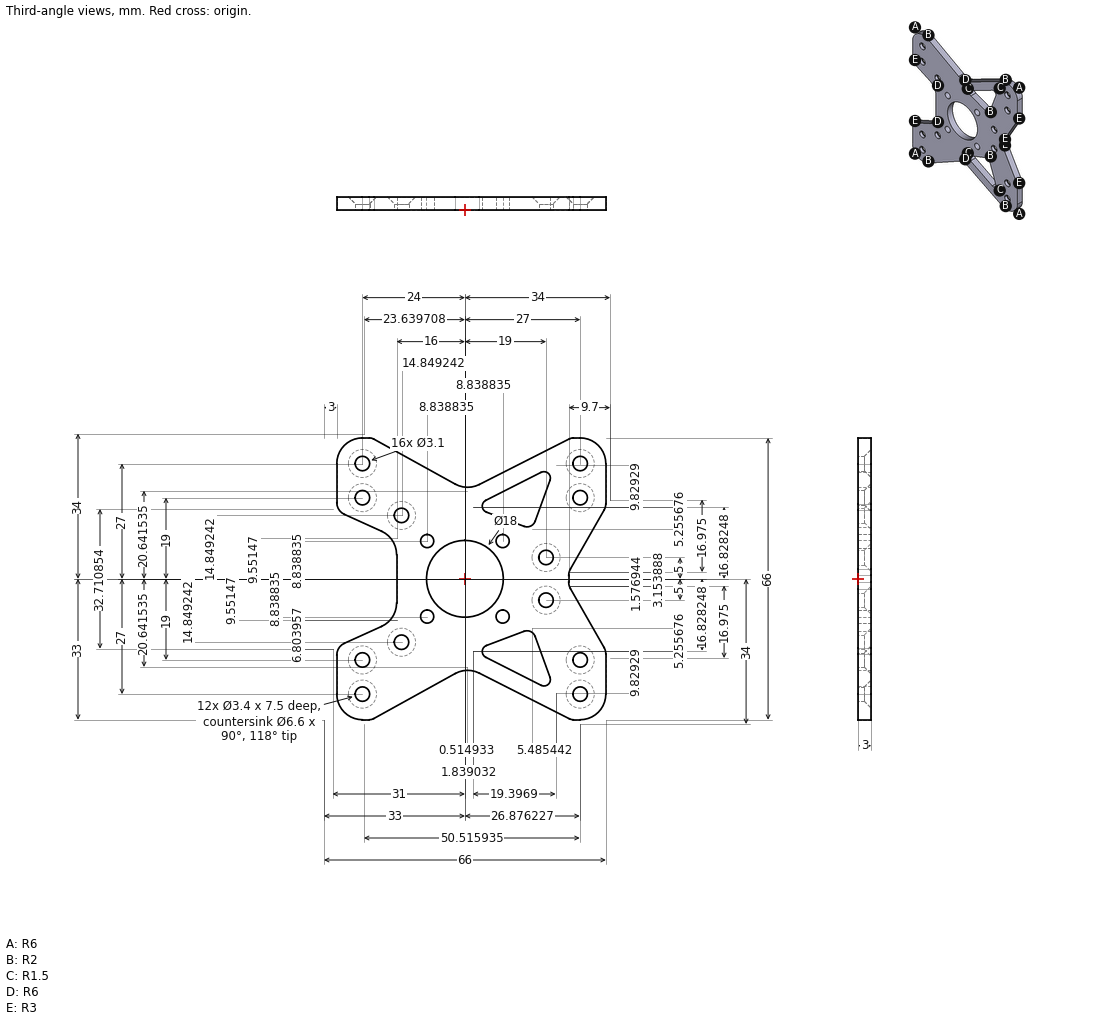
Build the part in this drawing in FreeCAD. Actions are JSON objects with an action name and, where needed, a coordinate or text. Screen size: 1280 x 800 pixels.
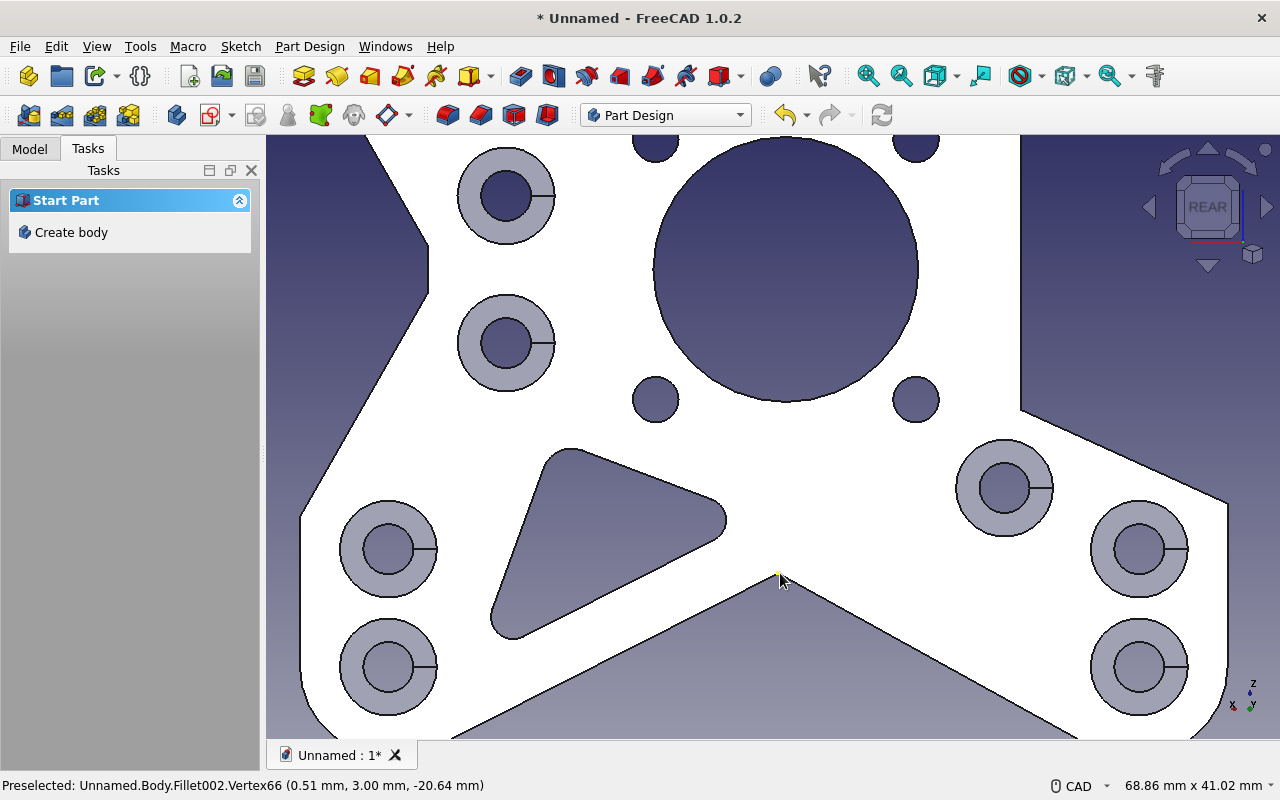
{"action": "key", "text": "v f"}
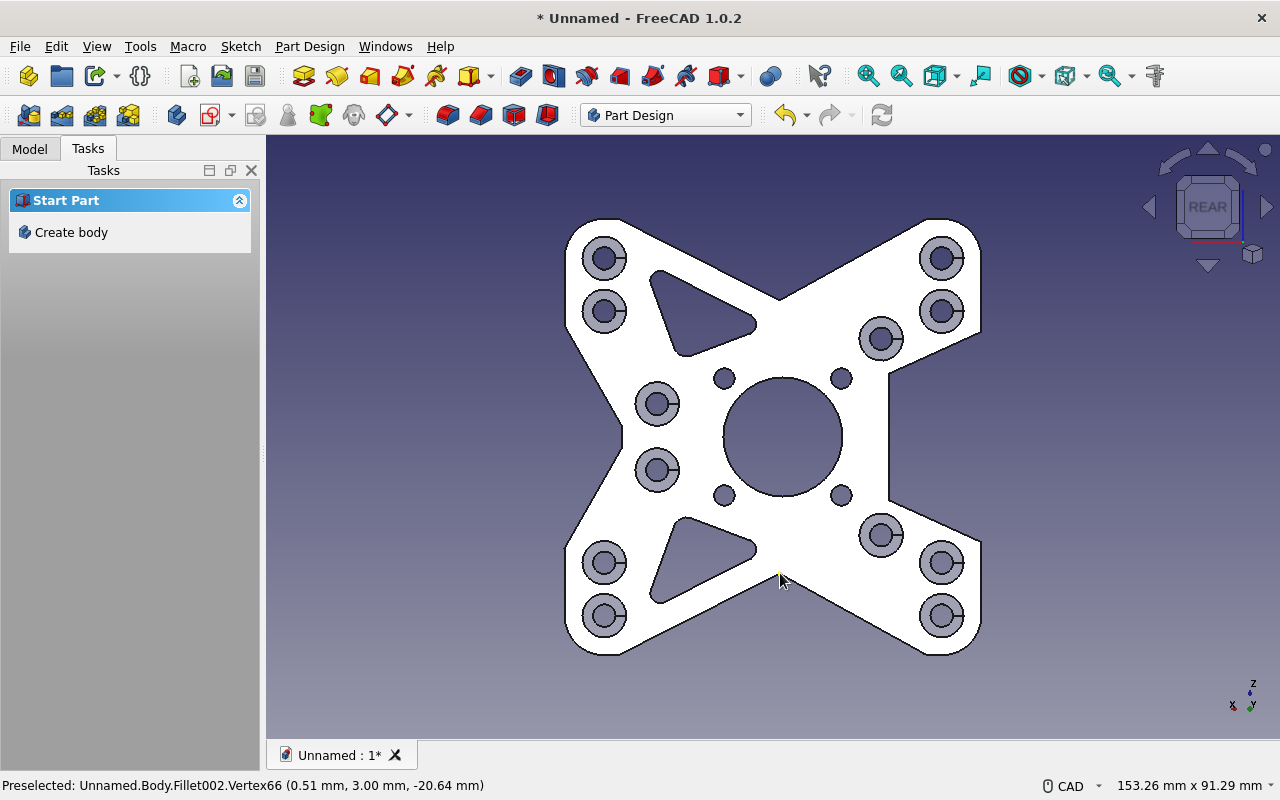
{"action": "key", "text": "6"}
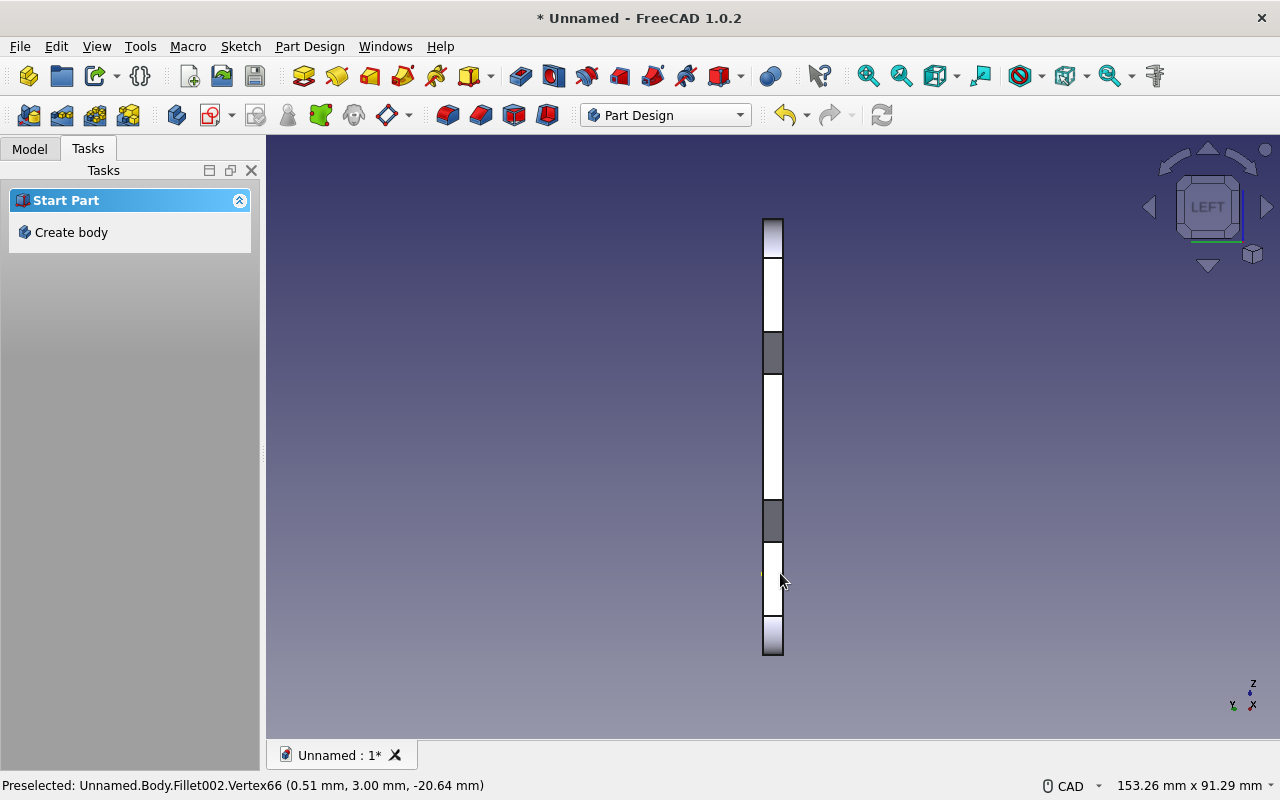
{"action": "scroll", "coordinate": [773, 573], "scroll_direction": "up", "scroll_amount": 4}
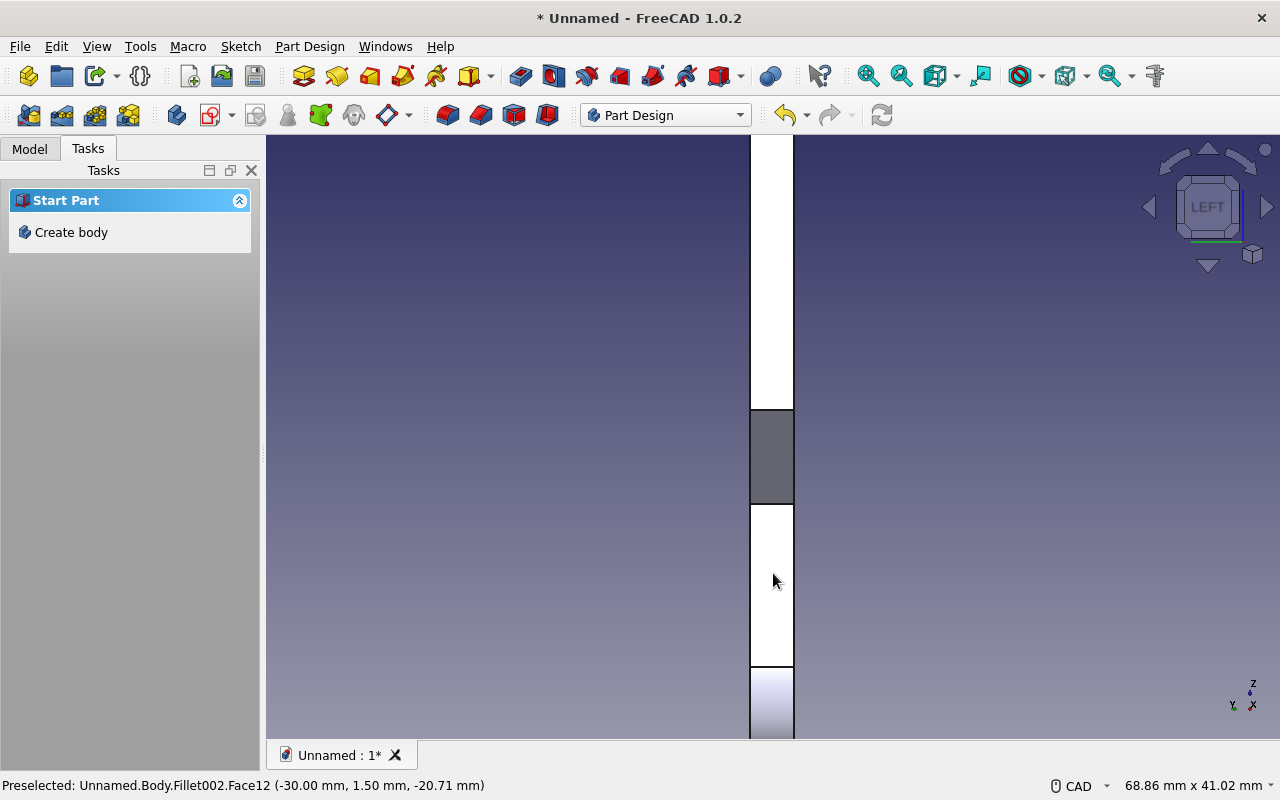
{"action": "left_click", "coordinate": [869, 76]}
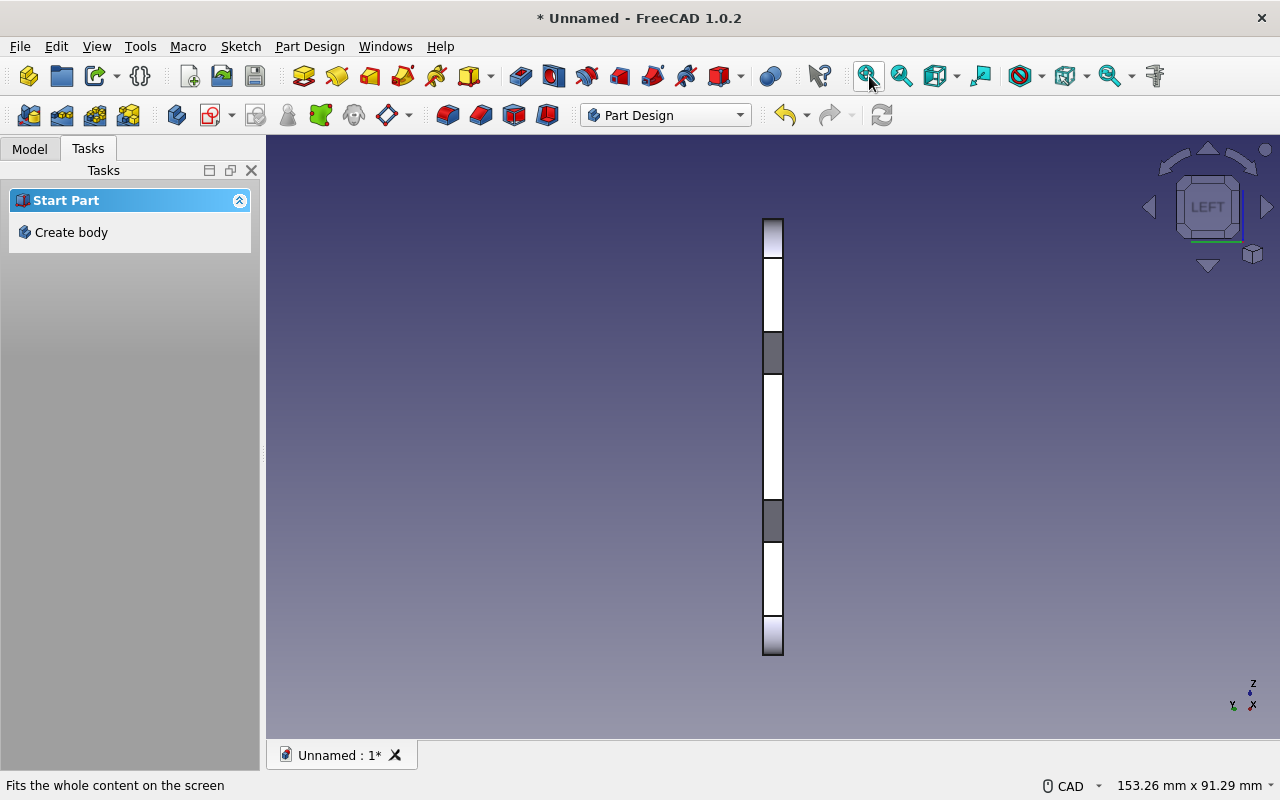
{"action": "key", "text": "v 3"}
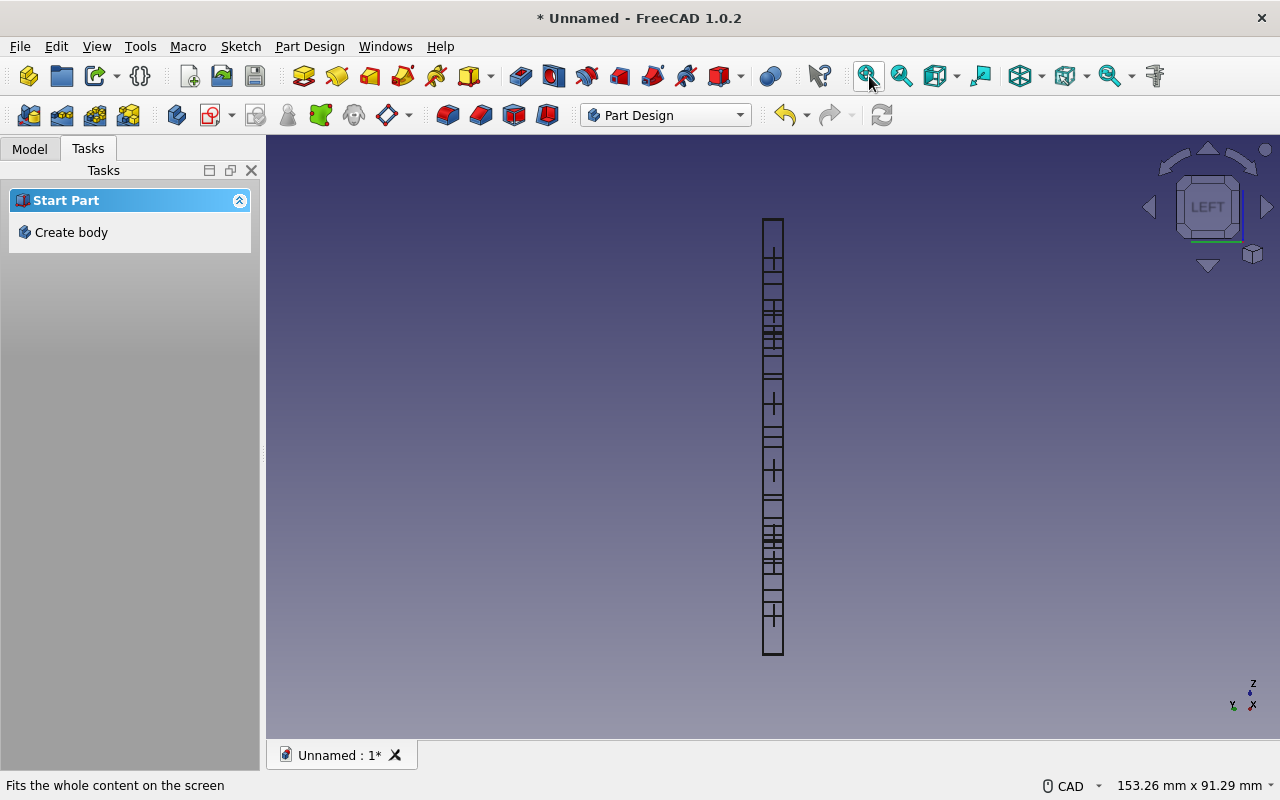
{"action": "key", "text": "0"}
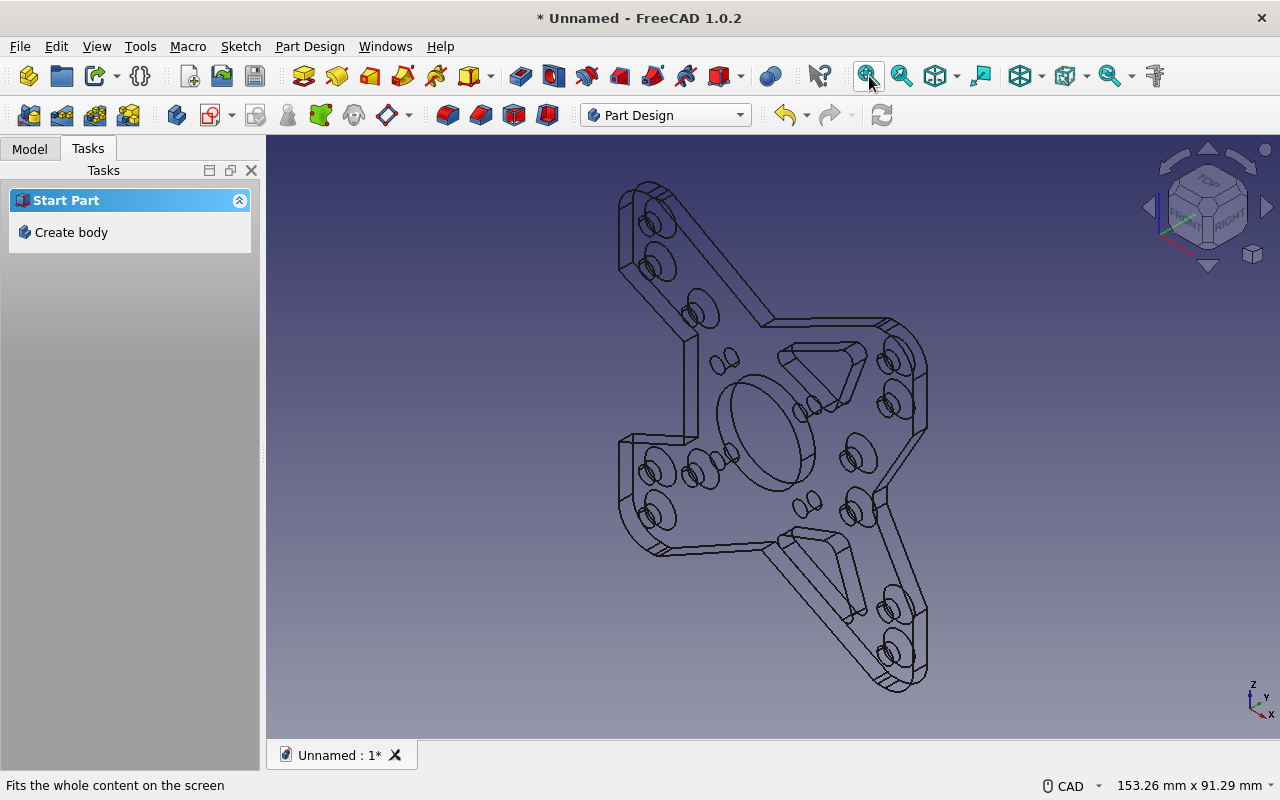
{"action": "left_click", "coordinate": [768, 545]}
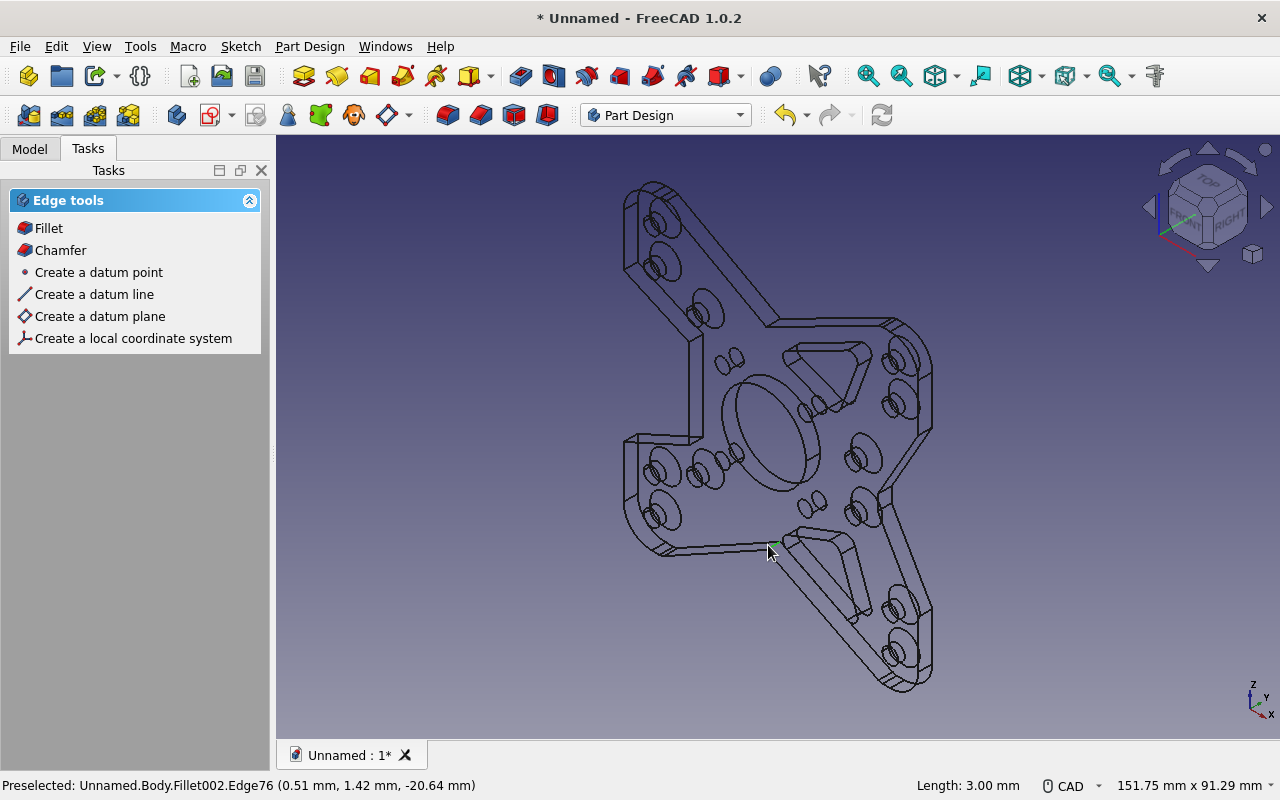
{"action": "left_click", "coordinate": [778, 319], "text": "ctrl"}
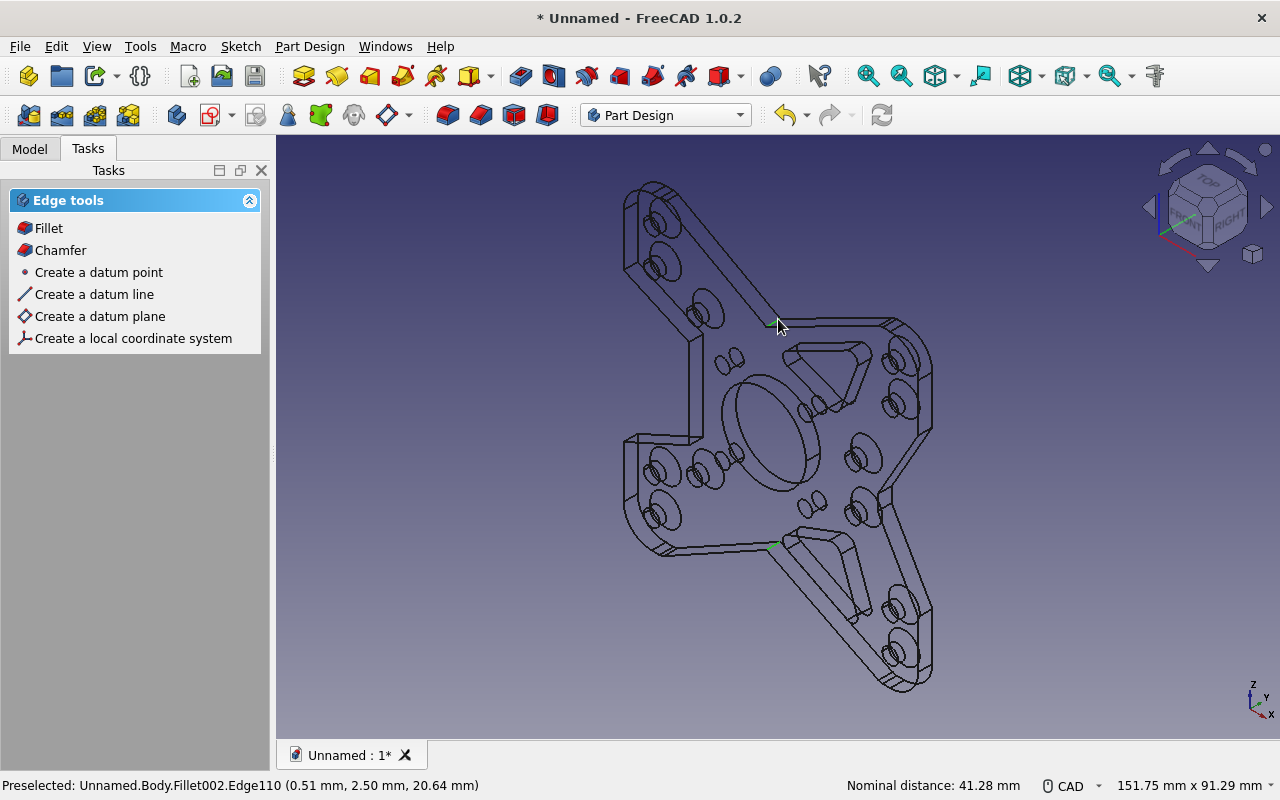
{"action": "left_click", "coordinate": [696, 337], "text": "ctrl"}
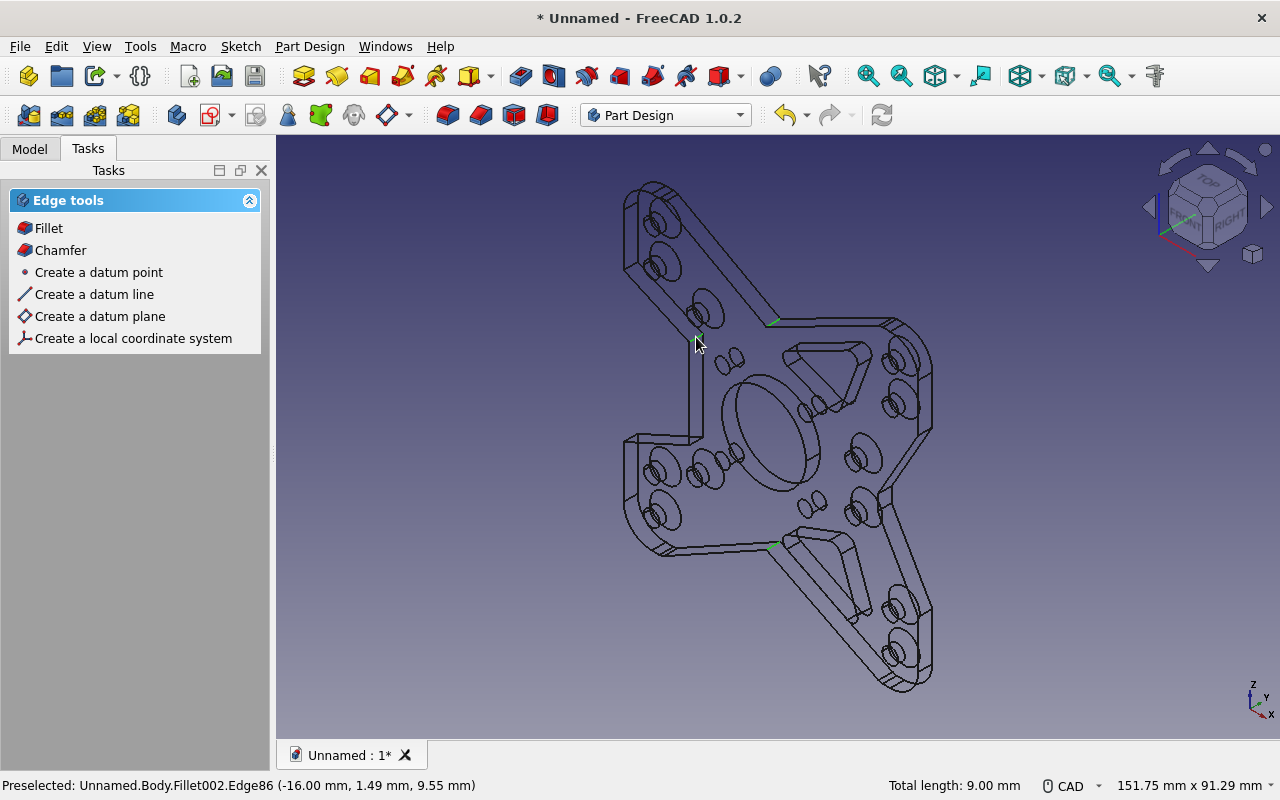
{"action": "left_click", "coordinate": [696, 440], "text": "ctrl"}